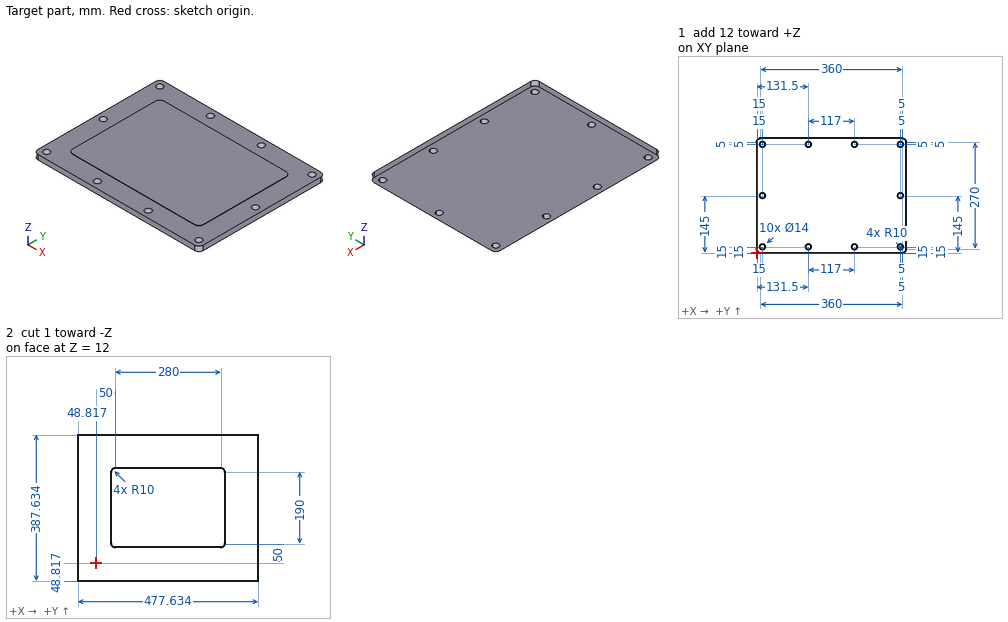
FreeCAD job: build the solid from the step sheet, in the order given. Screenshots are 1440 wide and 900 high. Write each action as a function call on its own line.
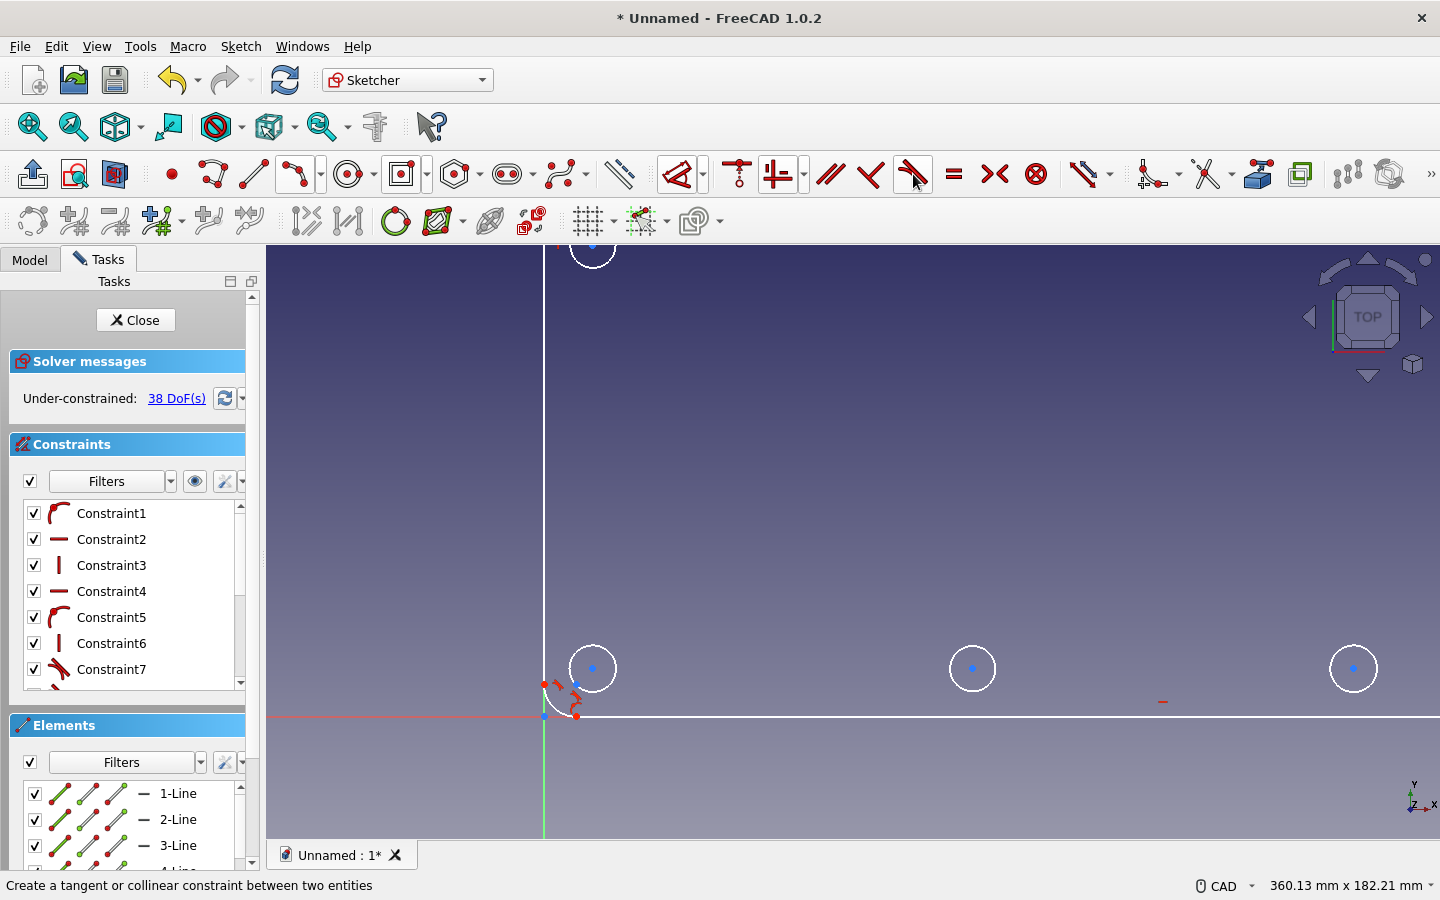
scroll(564, 715, down, 5)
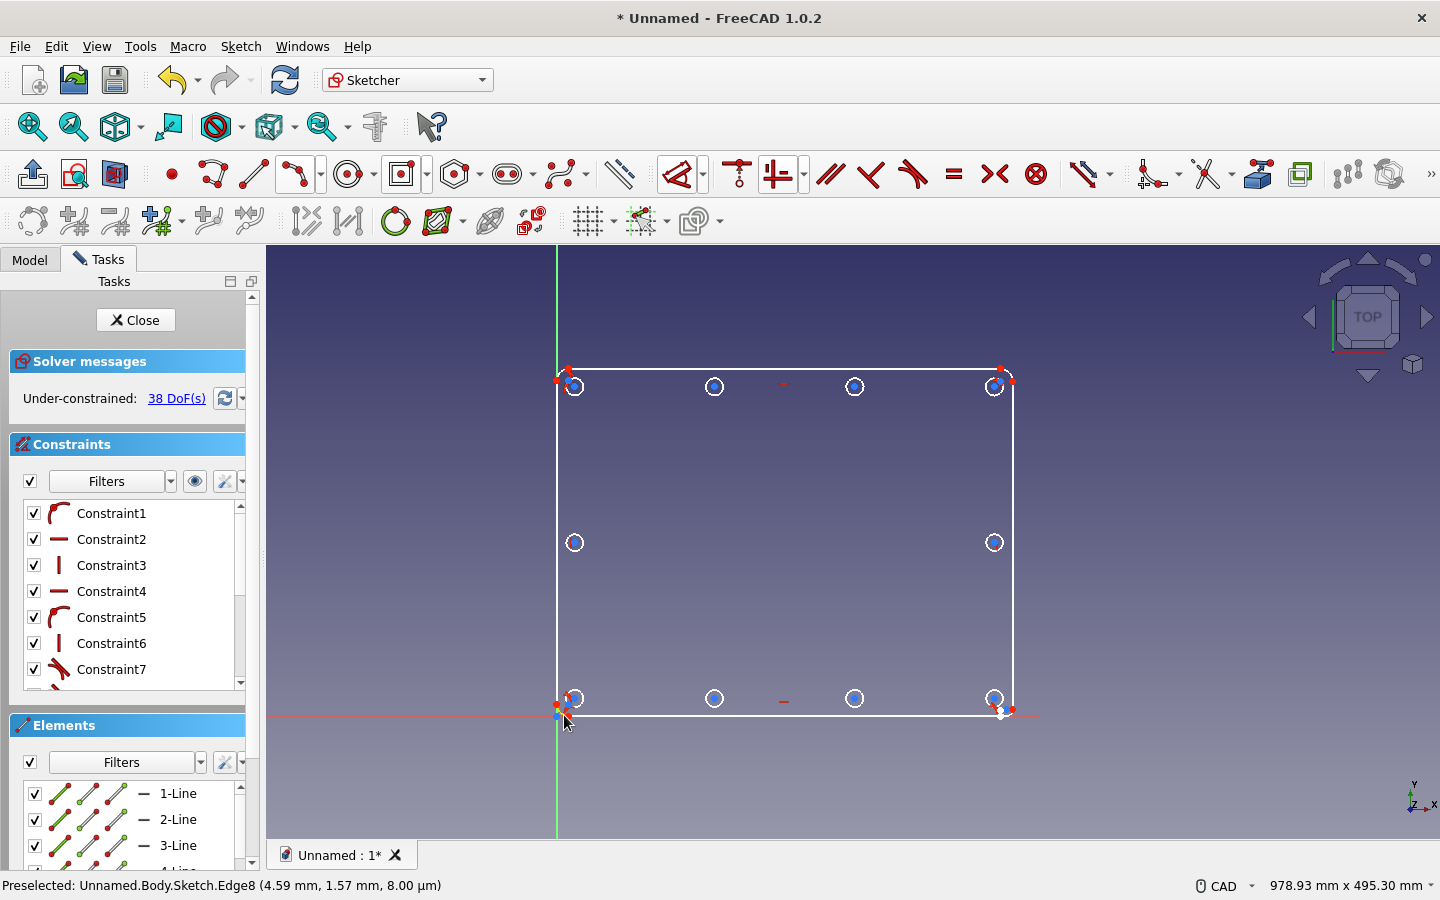
scroll(1010, 715, up, 5)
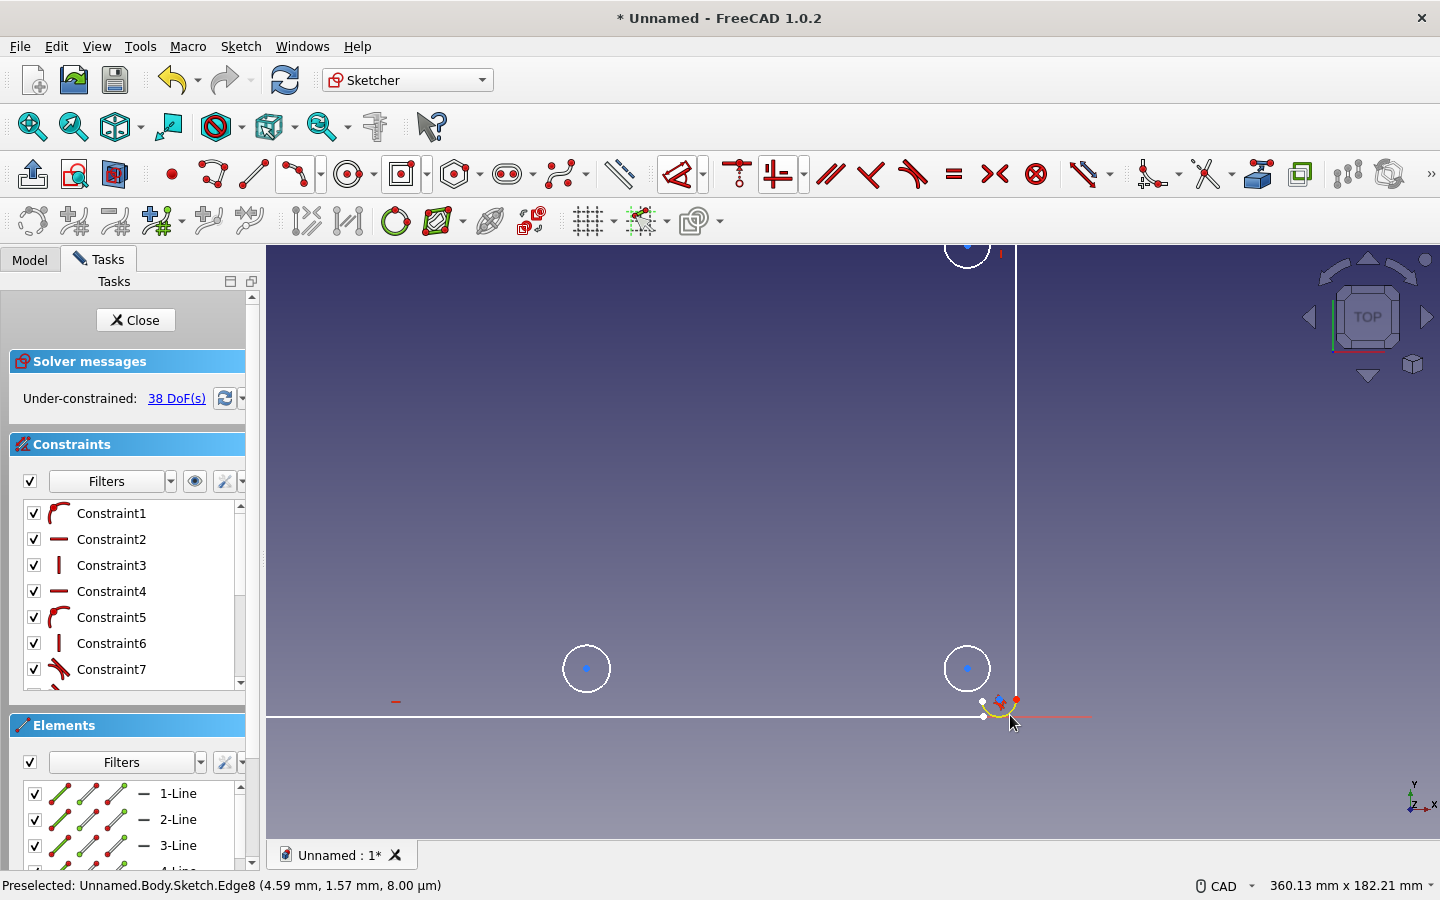
click(1010, 713)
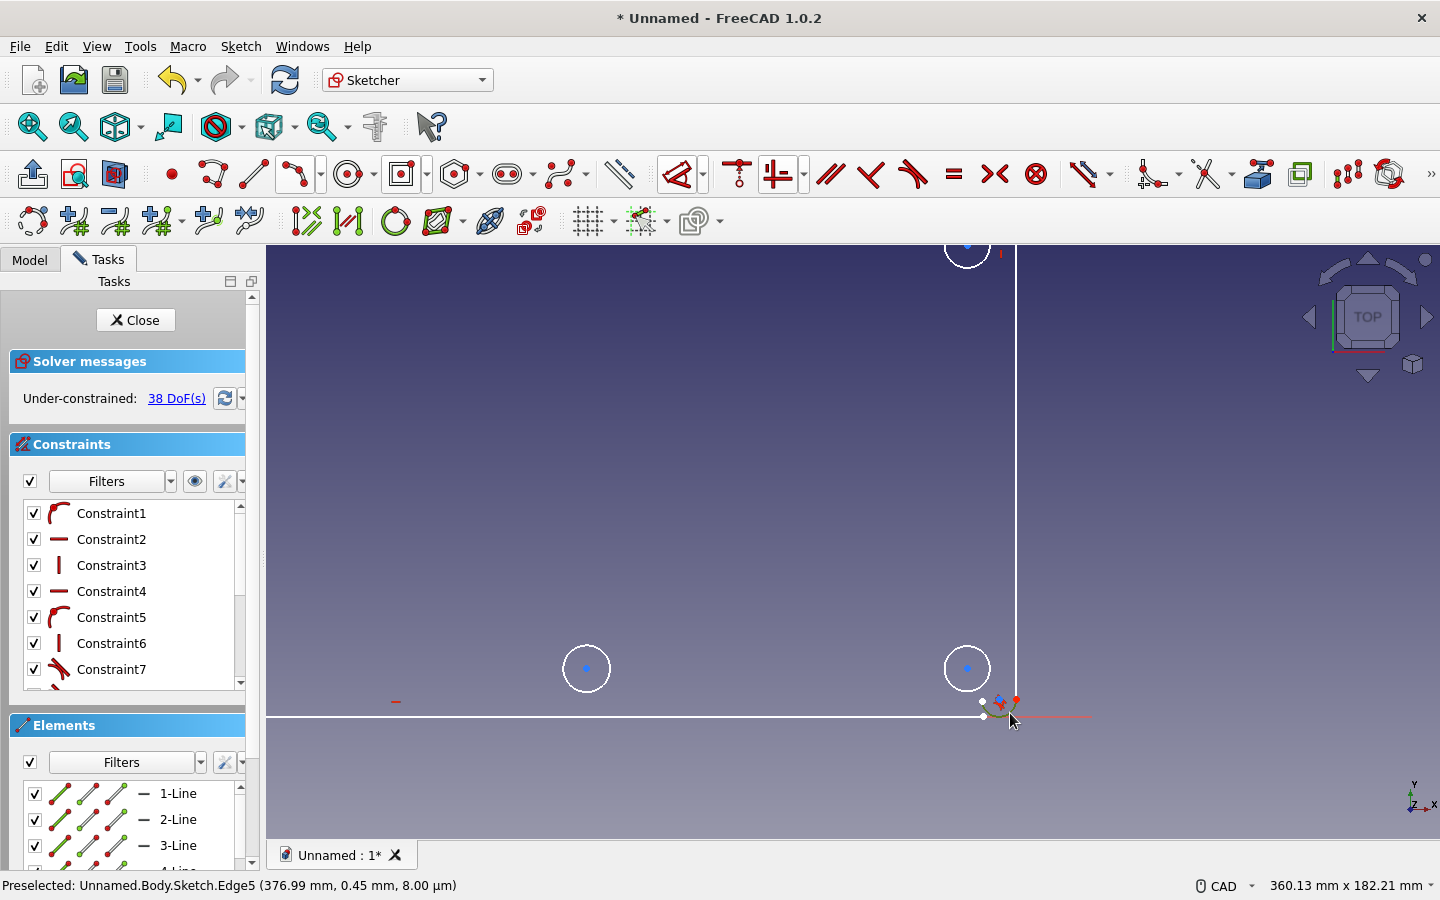
scroll(1010, 715, down, 5)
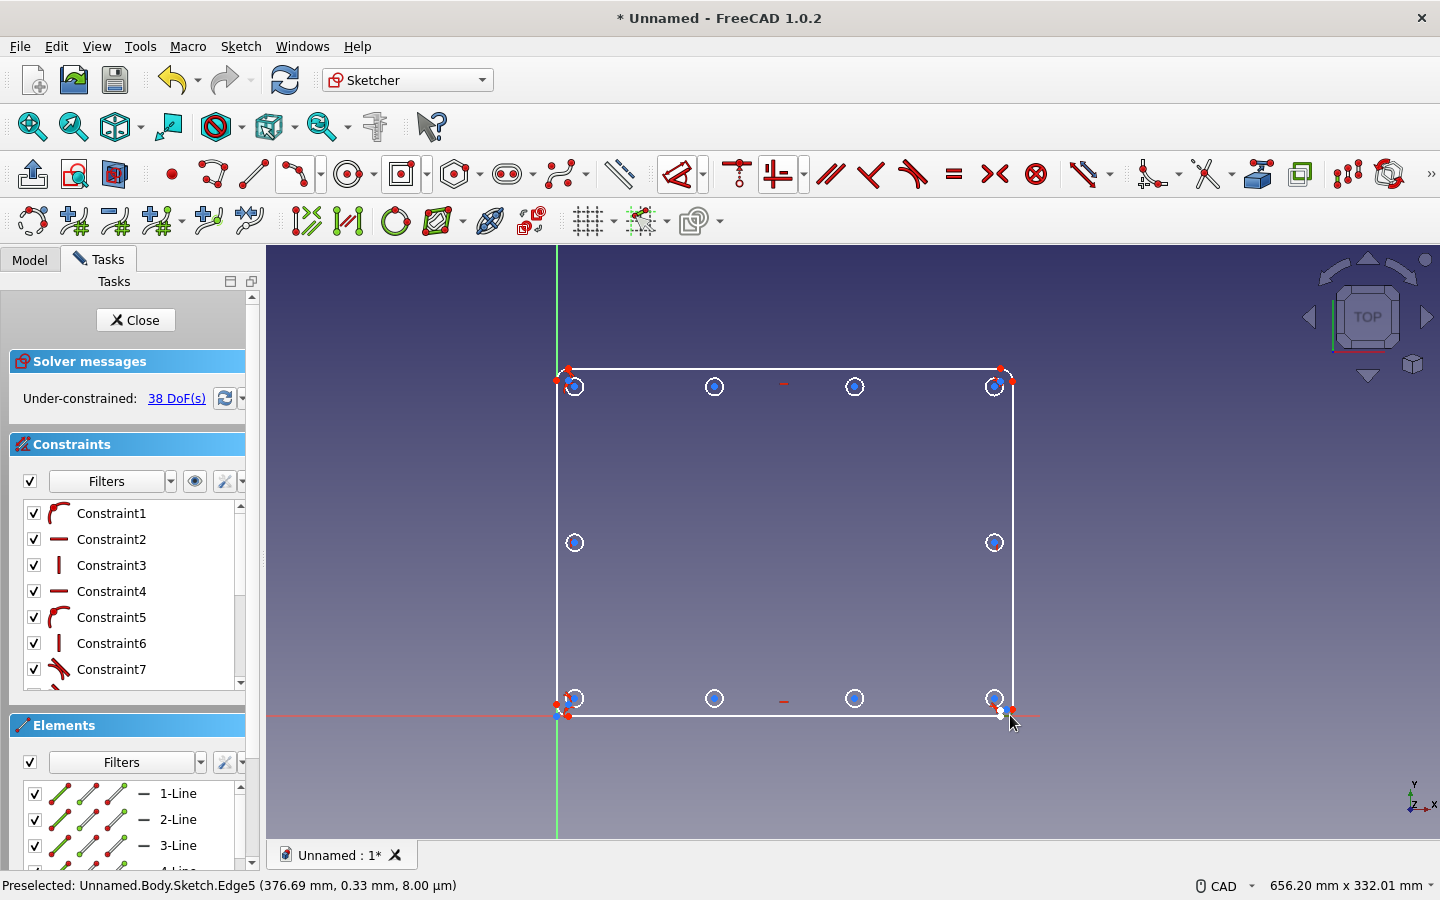
scroll(1011, 376, up, 5)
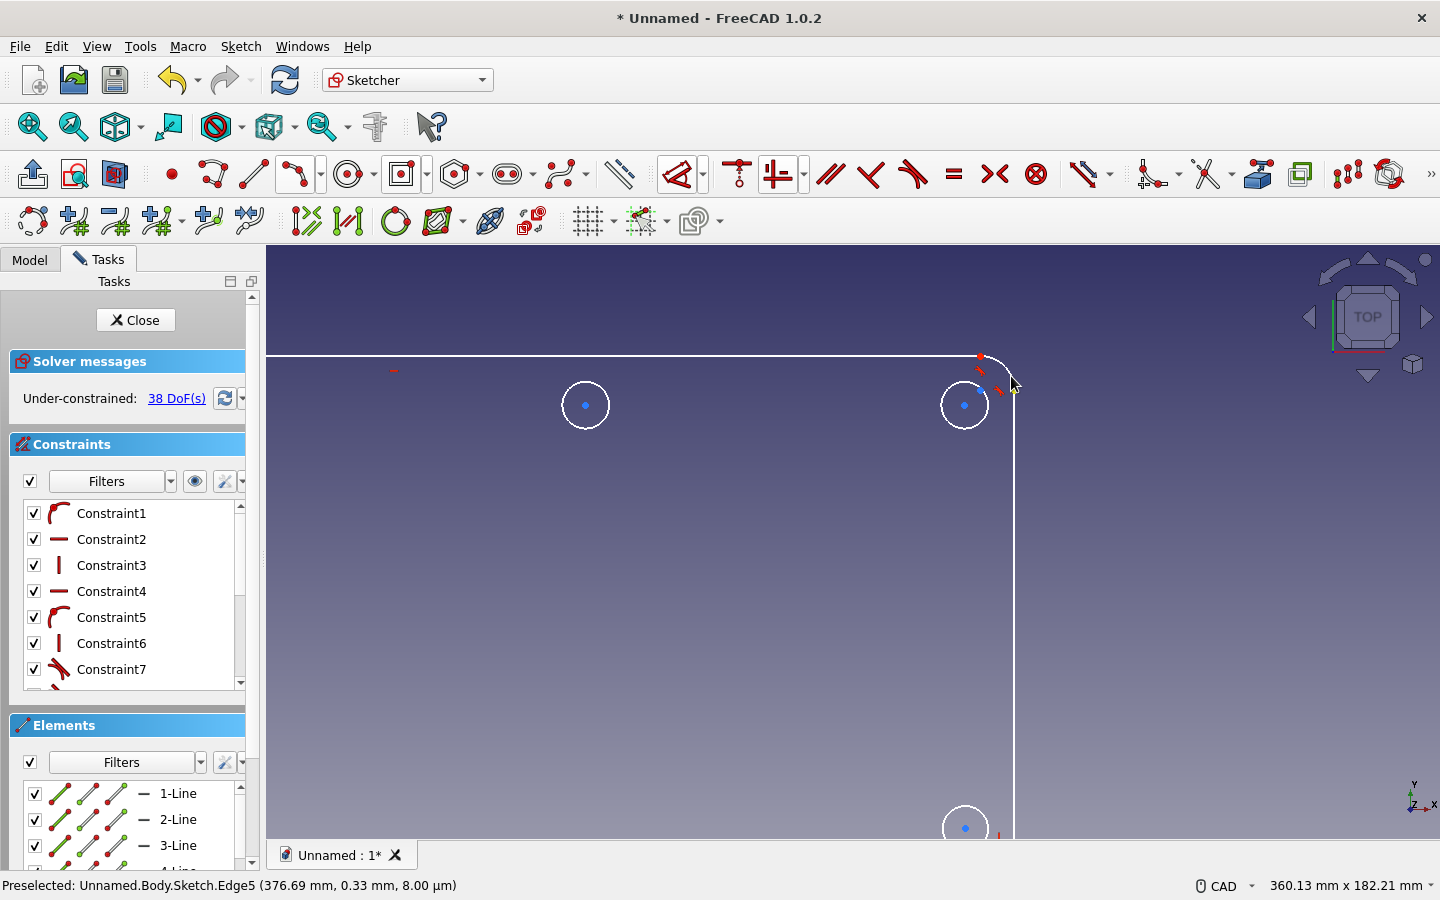
click(1011, 375)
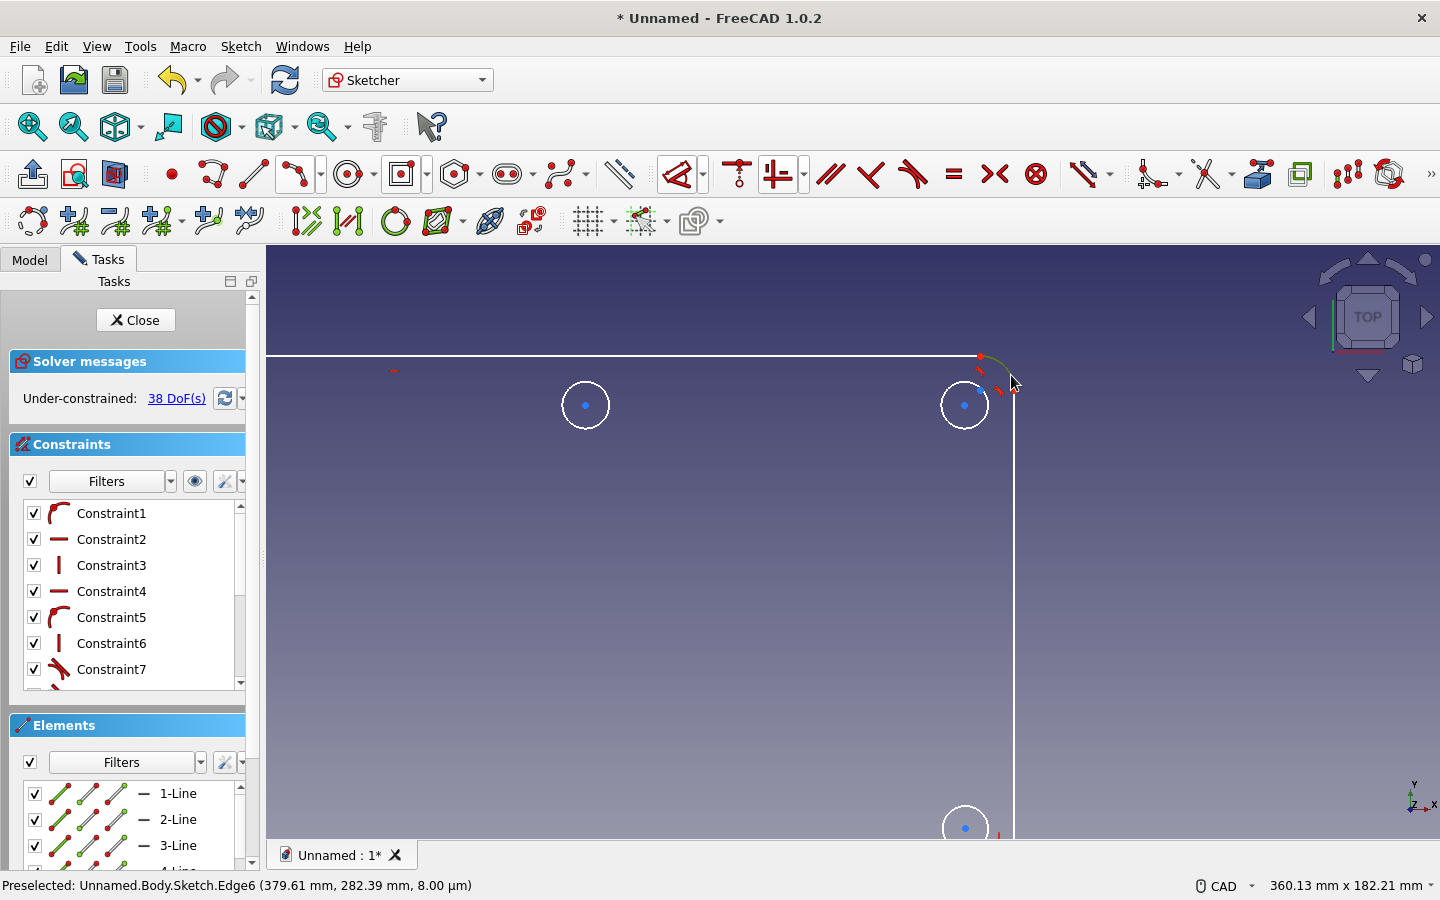
scroll(1011, 376, down, 5)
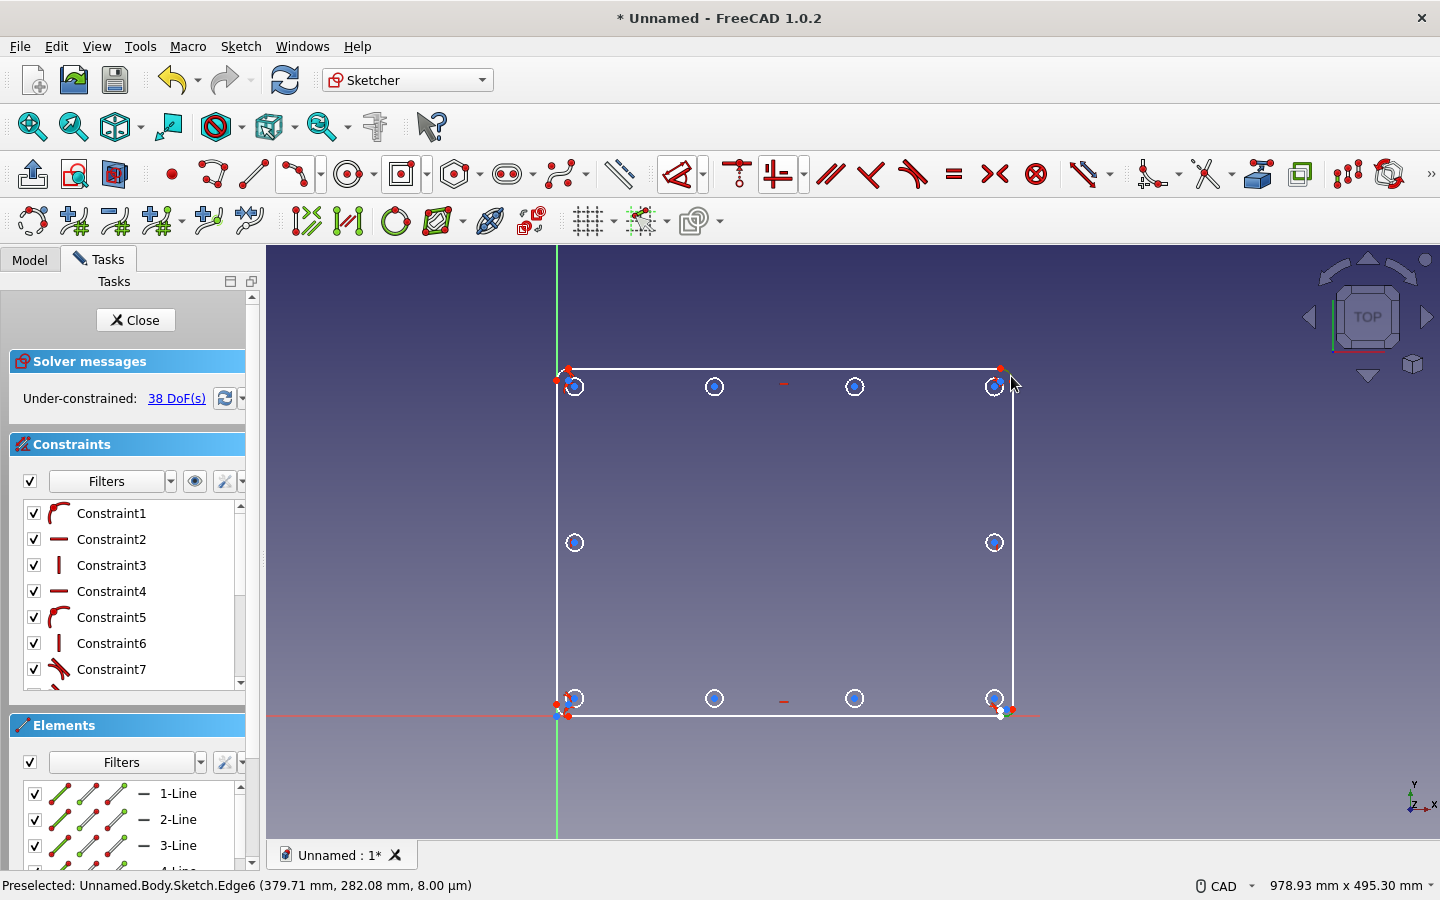
scroll(563, 370, up, 5)